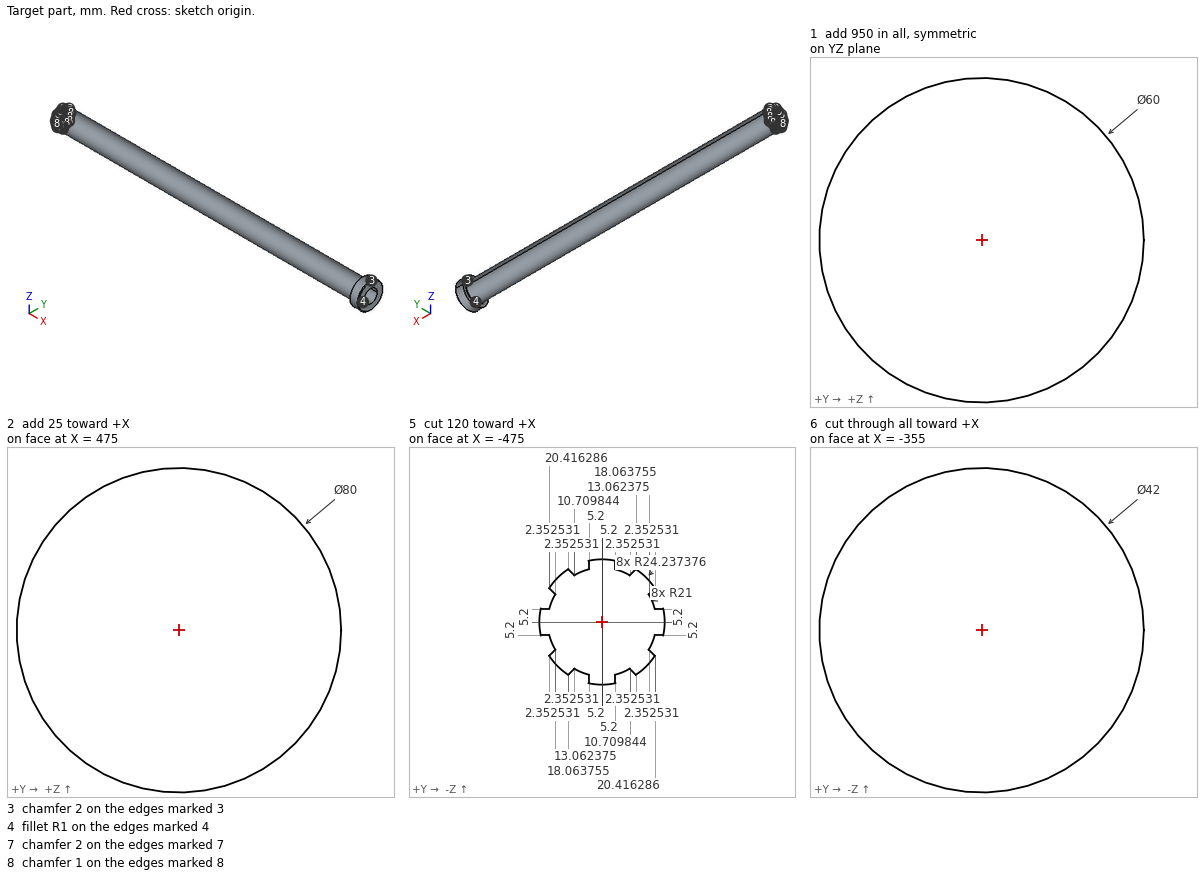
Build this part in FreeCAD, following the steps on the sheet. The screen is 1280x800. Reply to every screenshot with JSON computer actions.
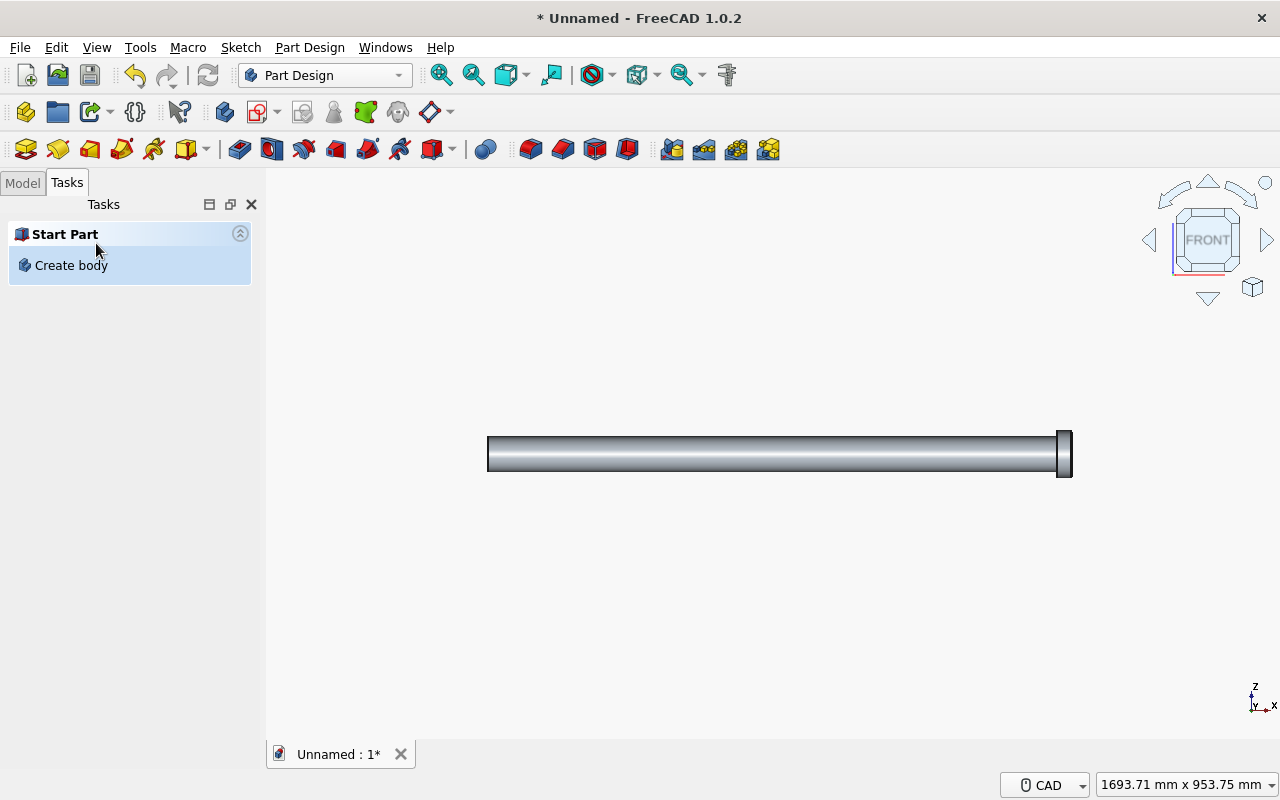
{"action": "key", "text": "3"}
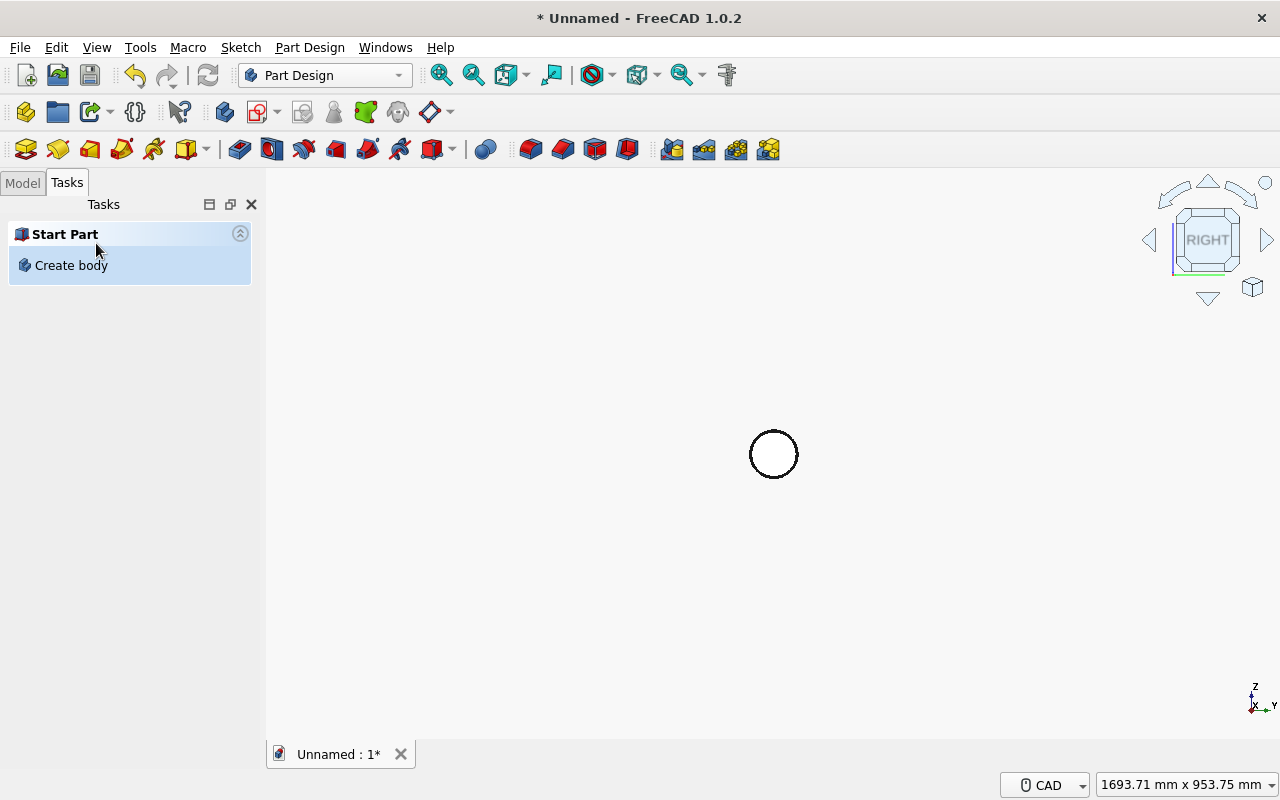
{"action": "left_click", "coordinate": [442, 76]}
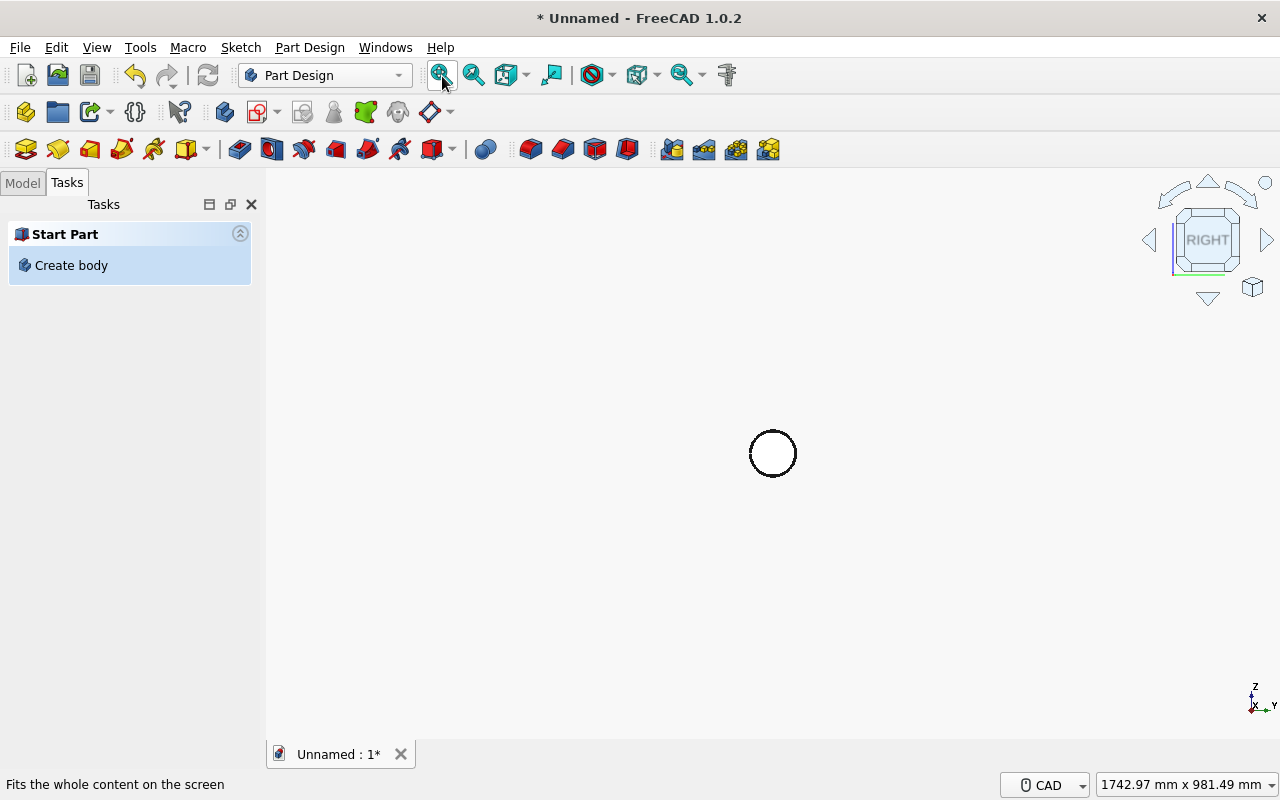
{"action": "key", "text": "5"}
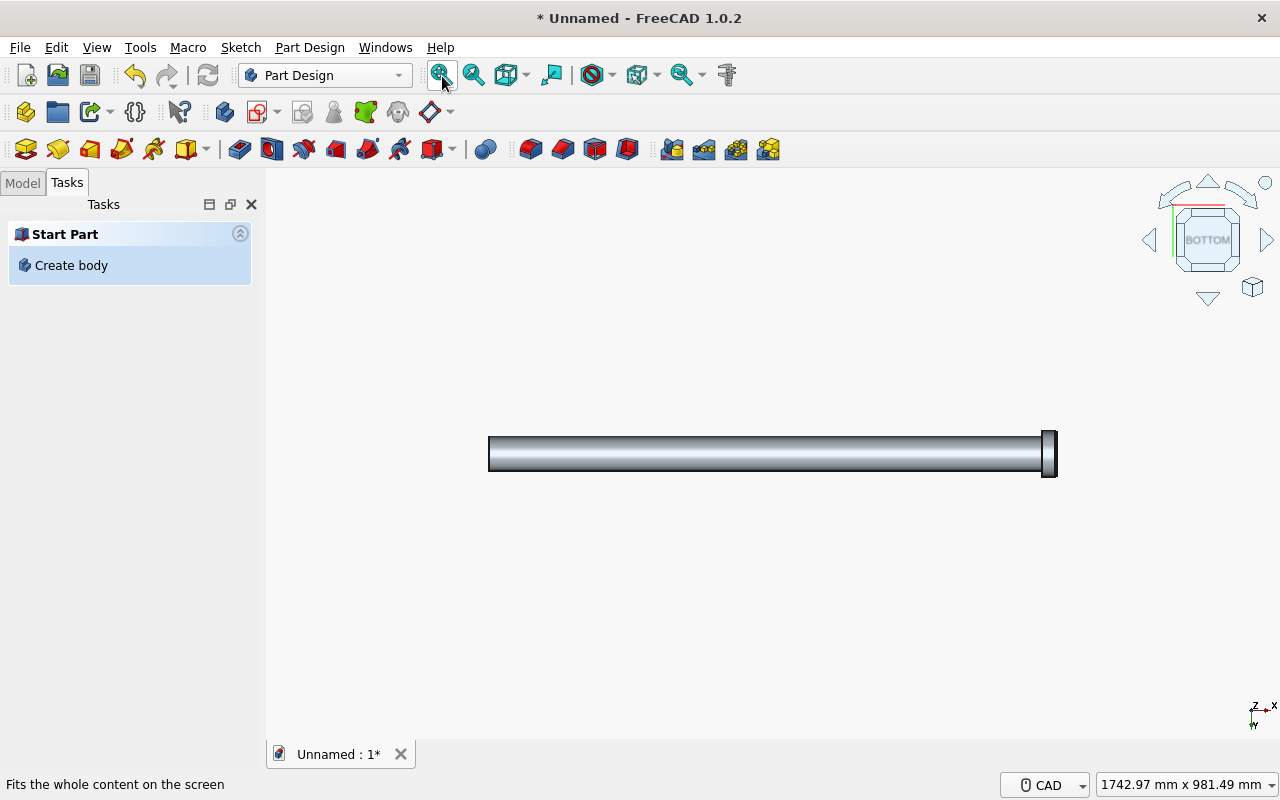
{"action": "key", "text": "4"}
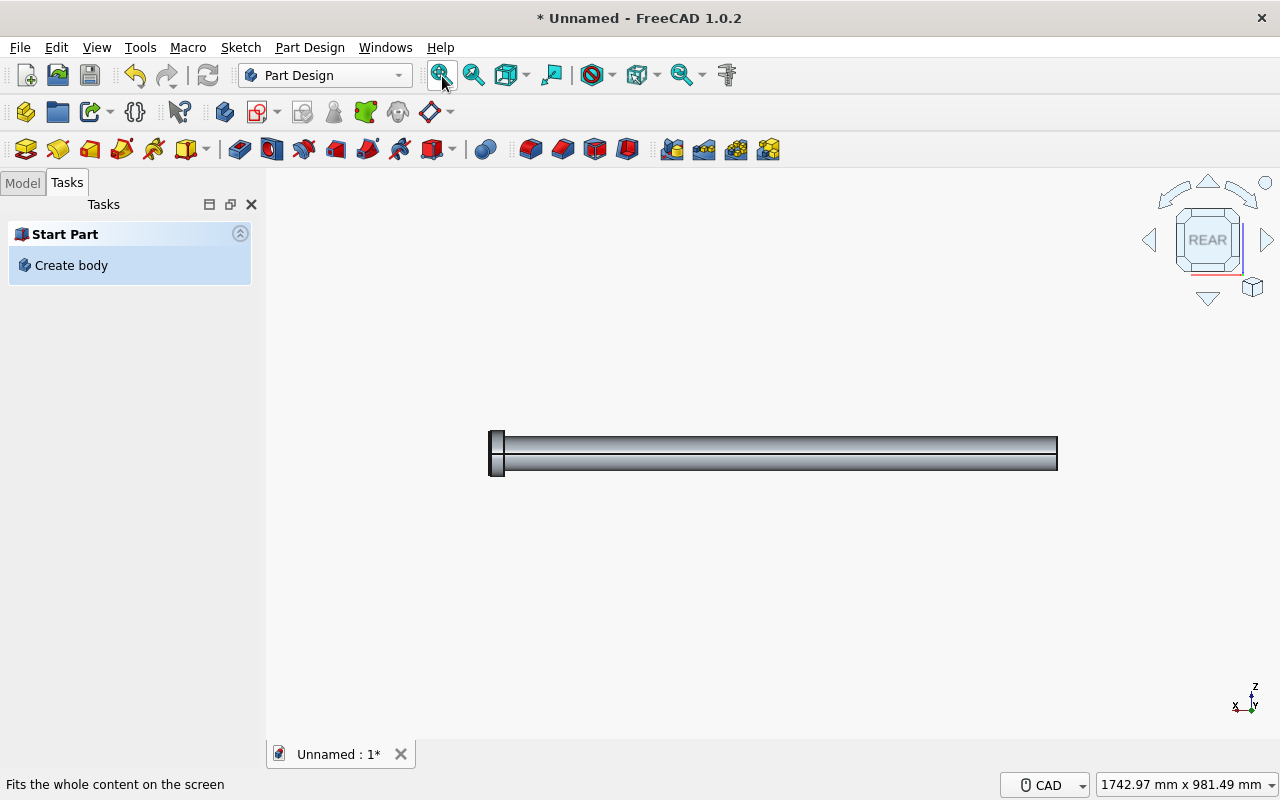
{"action": "key", "text": "6"}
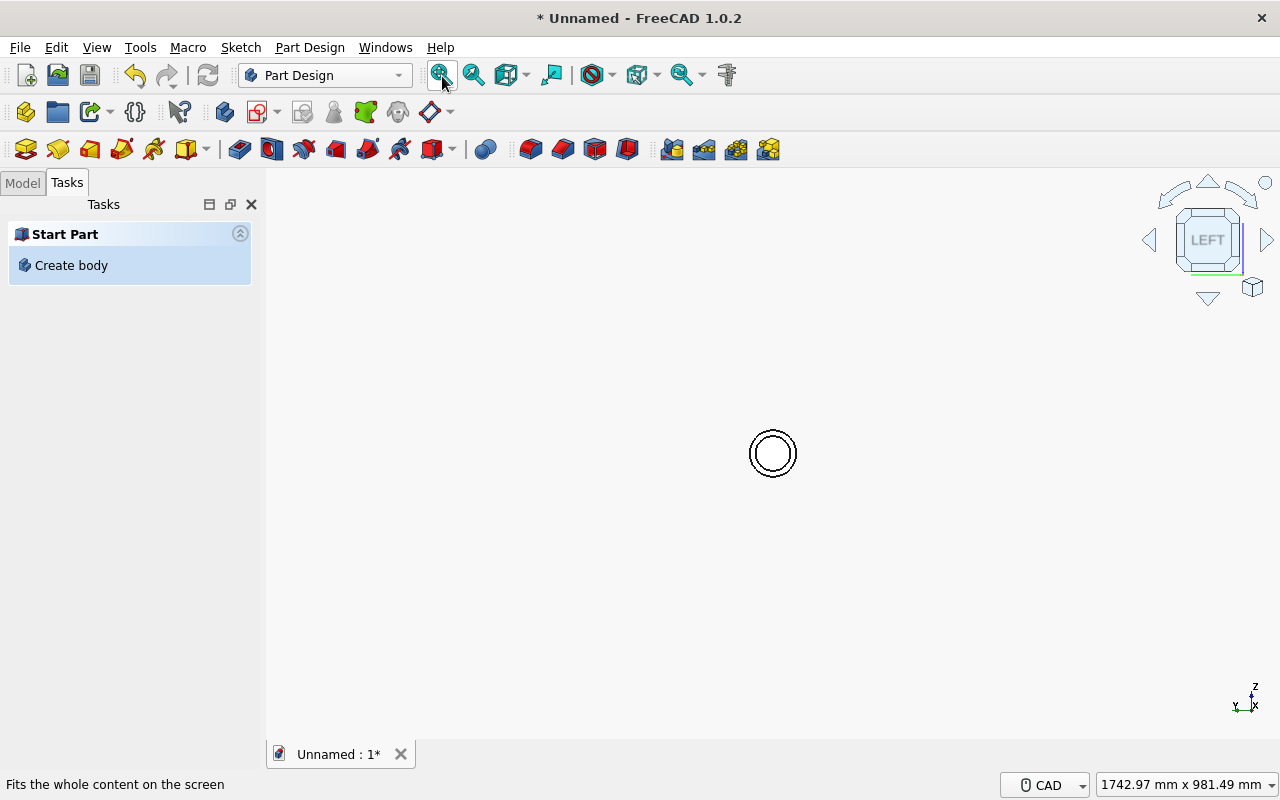
{"action": "left_click", "coordinate": [442, 76]}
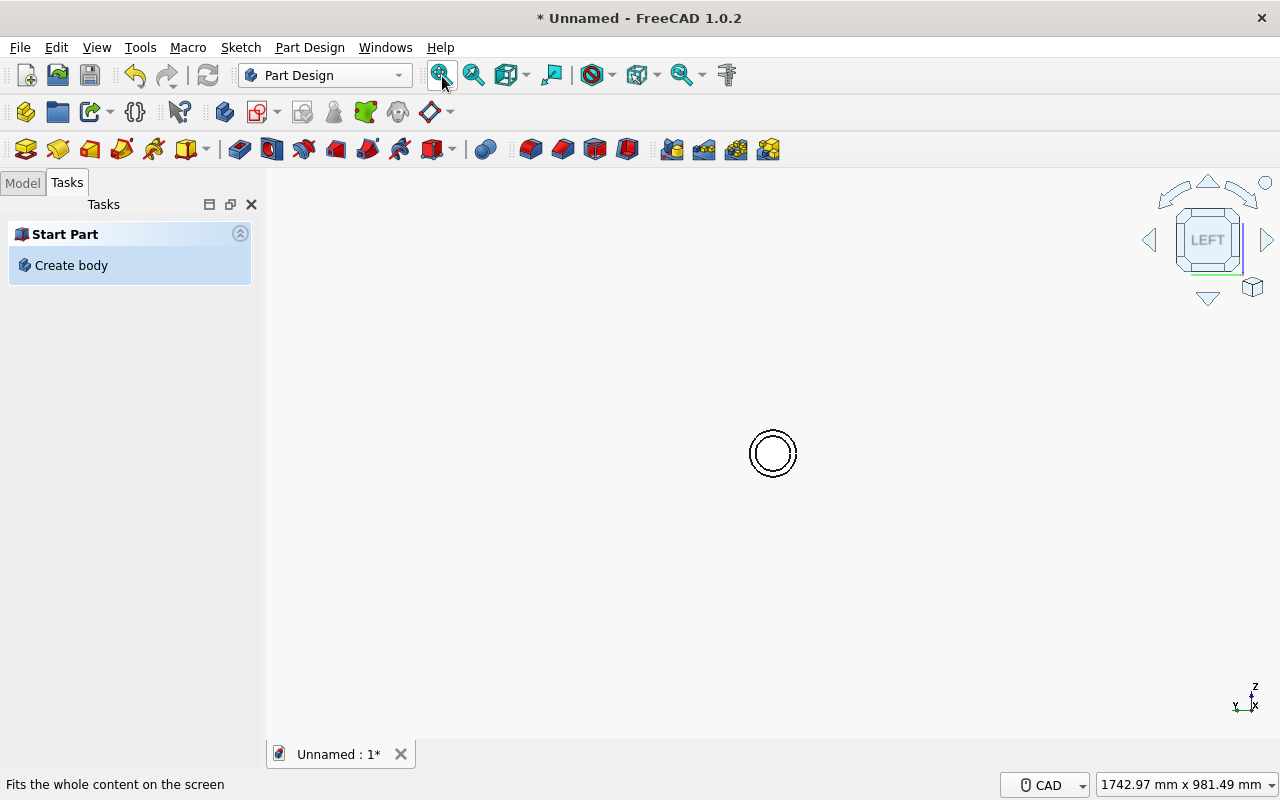
{"action": "key", "text": "v 3"}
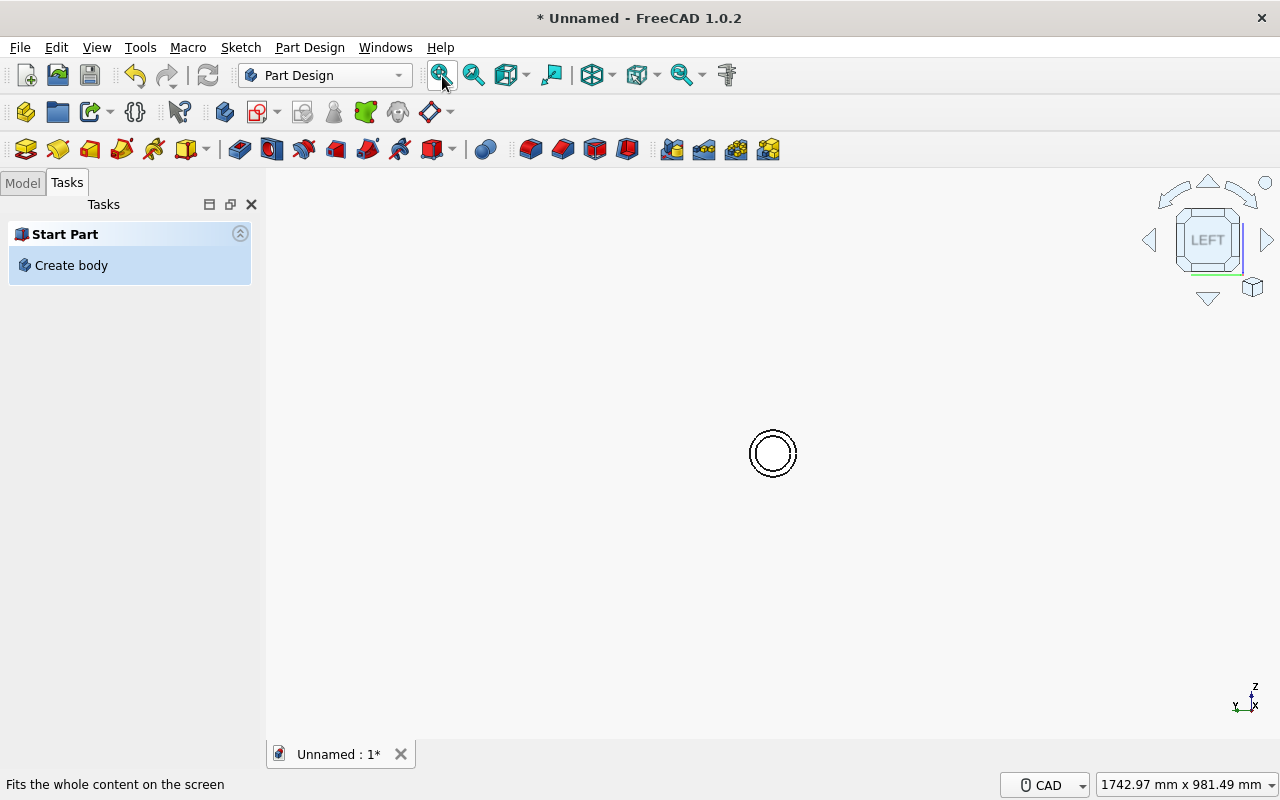
{"action": "key", "text": "0"}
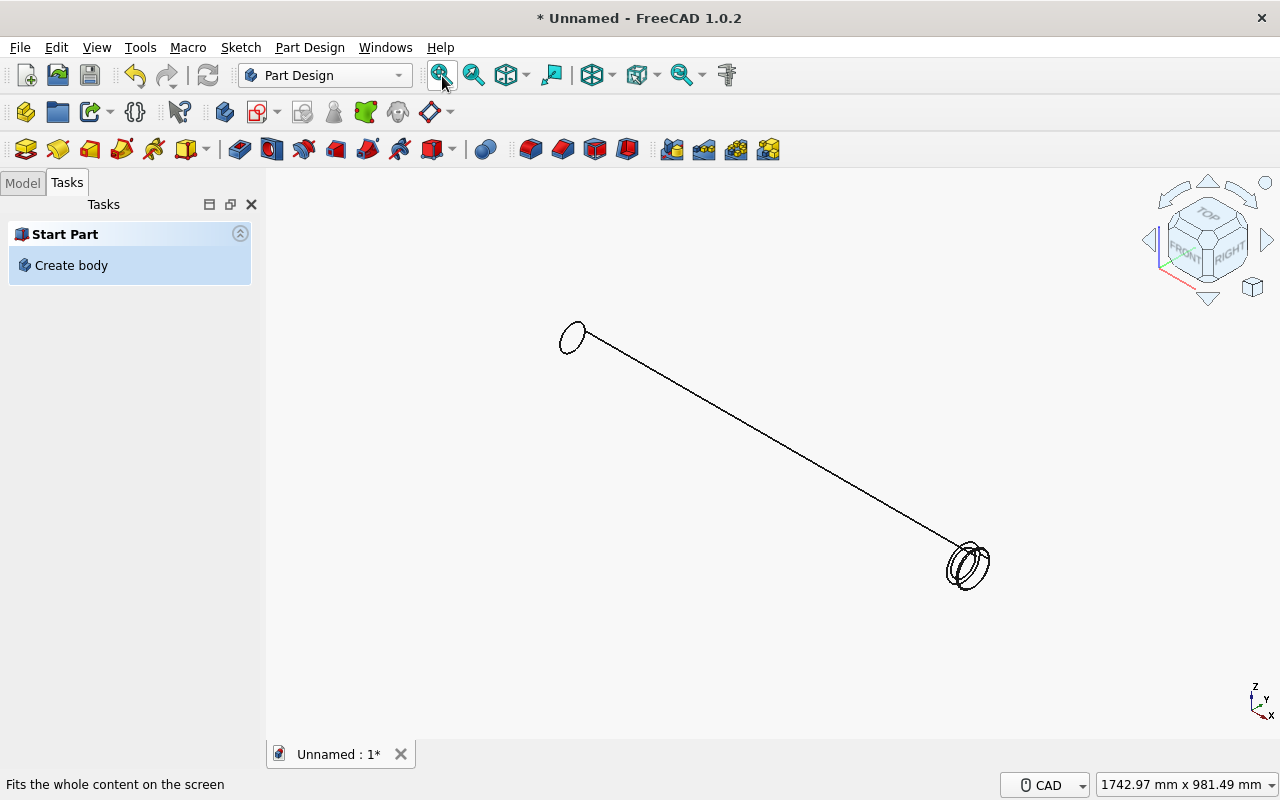
{"action": "left_click", "coordinate": [967, 574]}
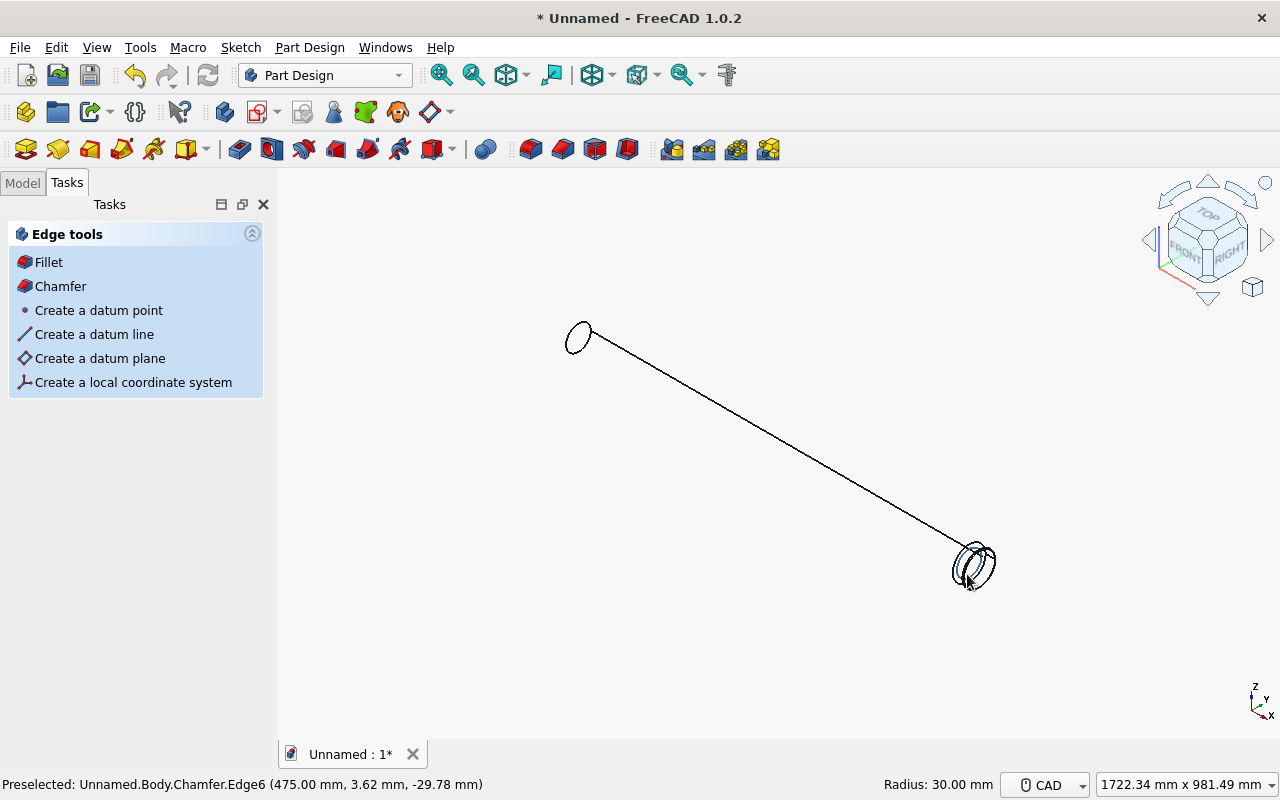
{"action": "key", "text": "v 1"}